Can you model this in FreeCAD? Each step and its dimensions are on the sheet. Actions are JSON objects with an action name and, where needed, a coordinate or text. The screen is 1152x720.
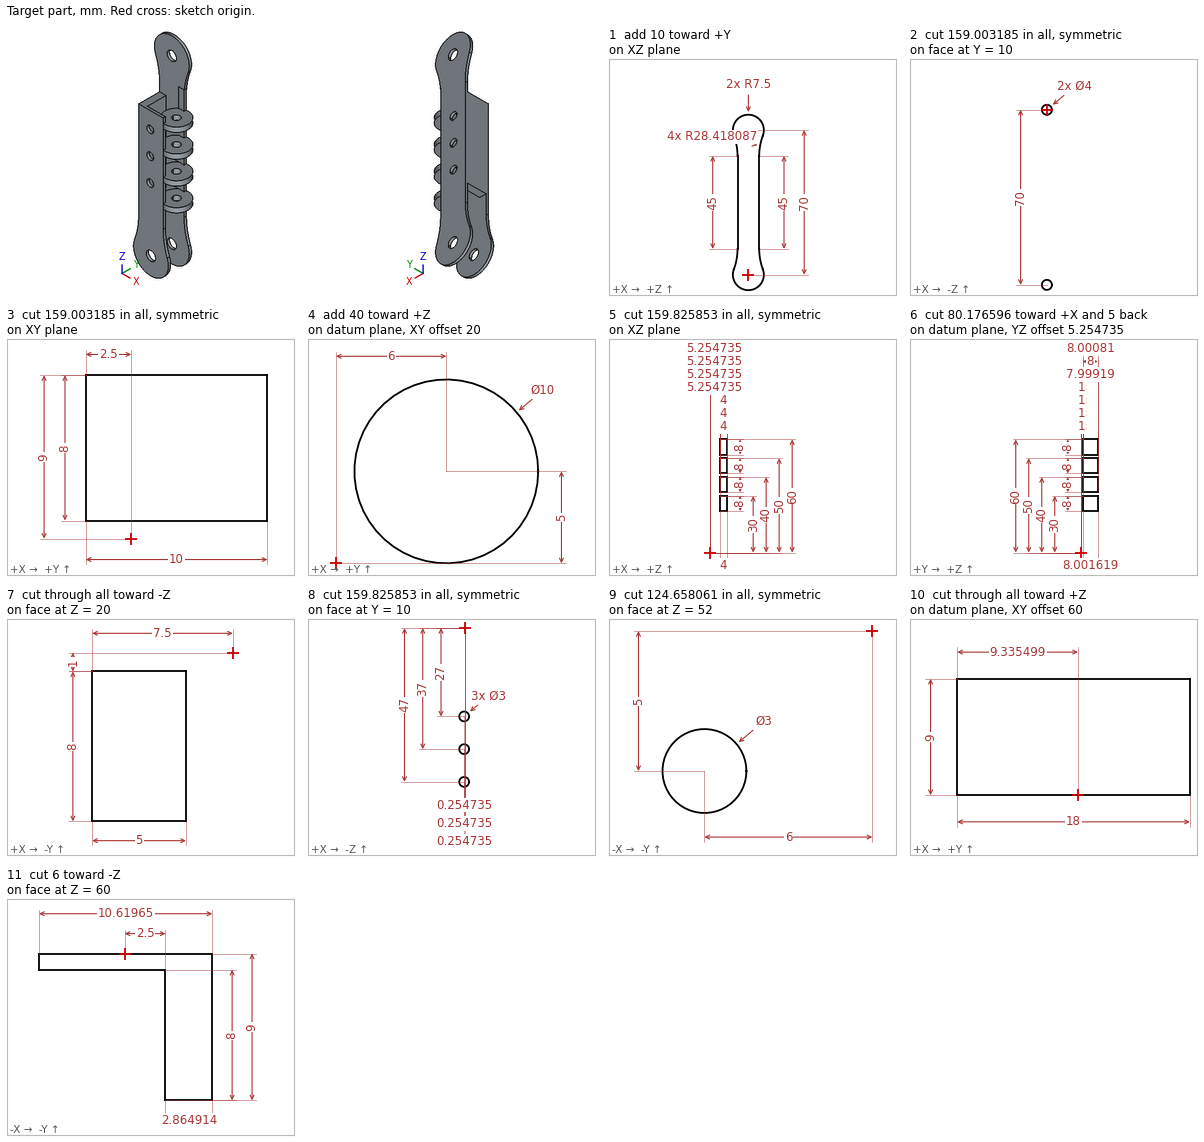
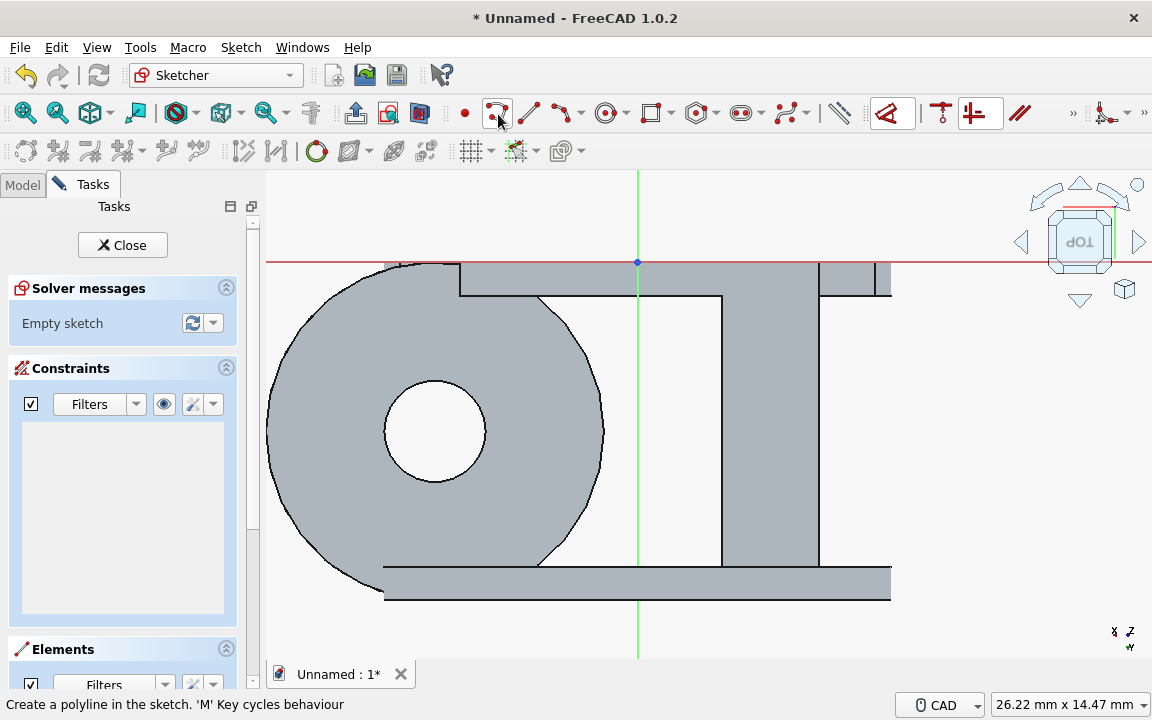
{"action": "left_click", "coordinate": [722, 296]}
{"action": "left_click", "coordinate": [722, 567]}
{"action": "left_click", "coordinate": [819, 567]}
{"action": "left_click", "coordinate": [819, 262]}
{"action": "left_click", "coordinate": [460, 271]}
{"action": "left_click", "coordinate": [460, 296]}
{"action": "left_click", "coordinate": [722, 297]}
{"action": "key", "text": "Escape"}
{"action": "key", "text": "Escape"}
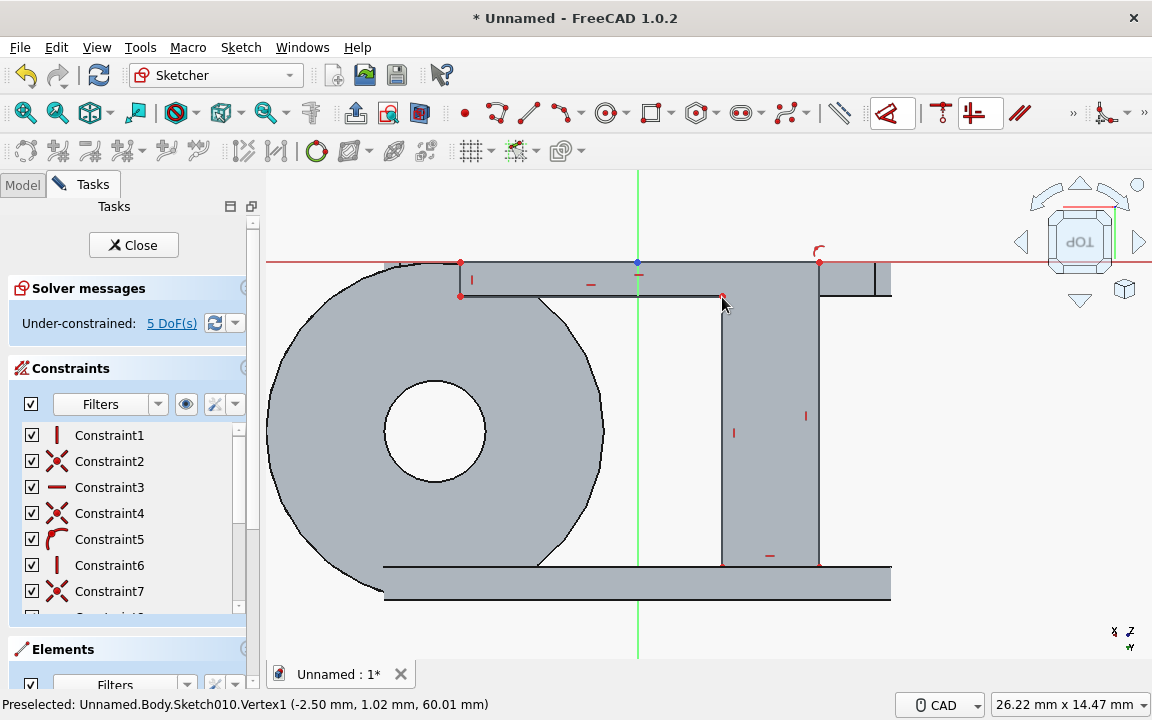
{"action": "left_click", "coordinate": [722, 378]}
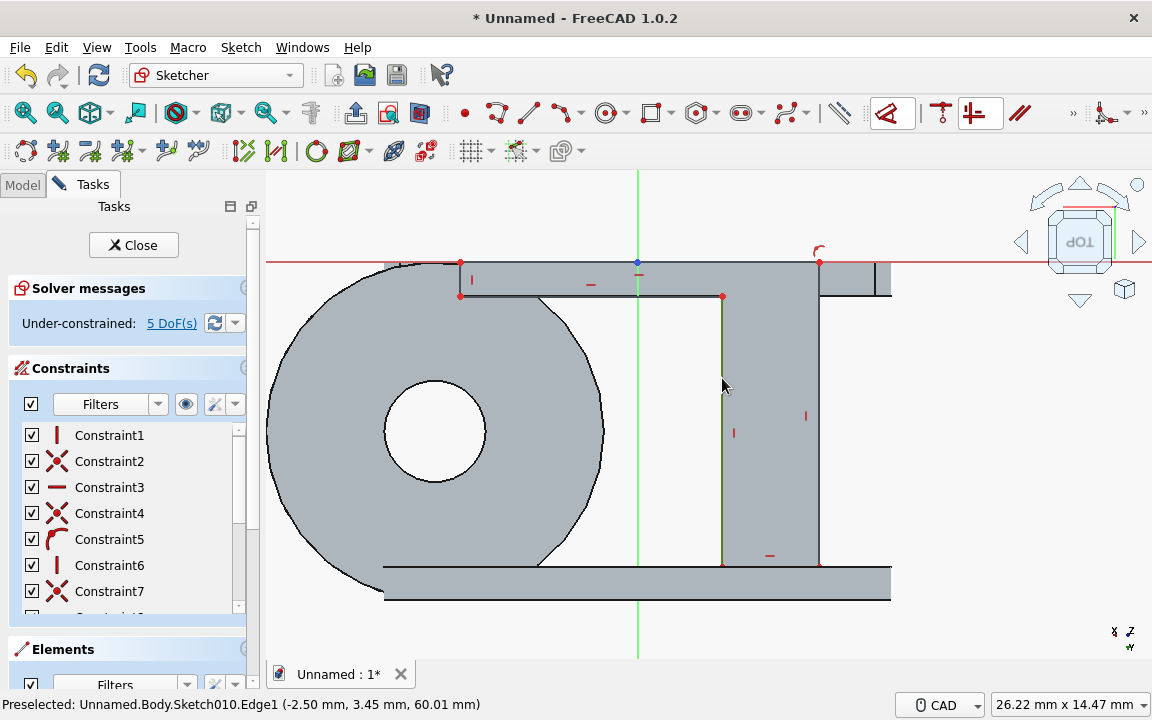
{"action": "left_click", "coordinate": [910, 114]}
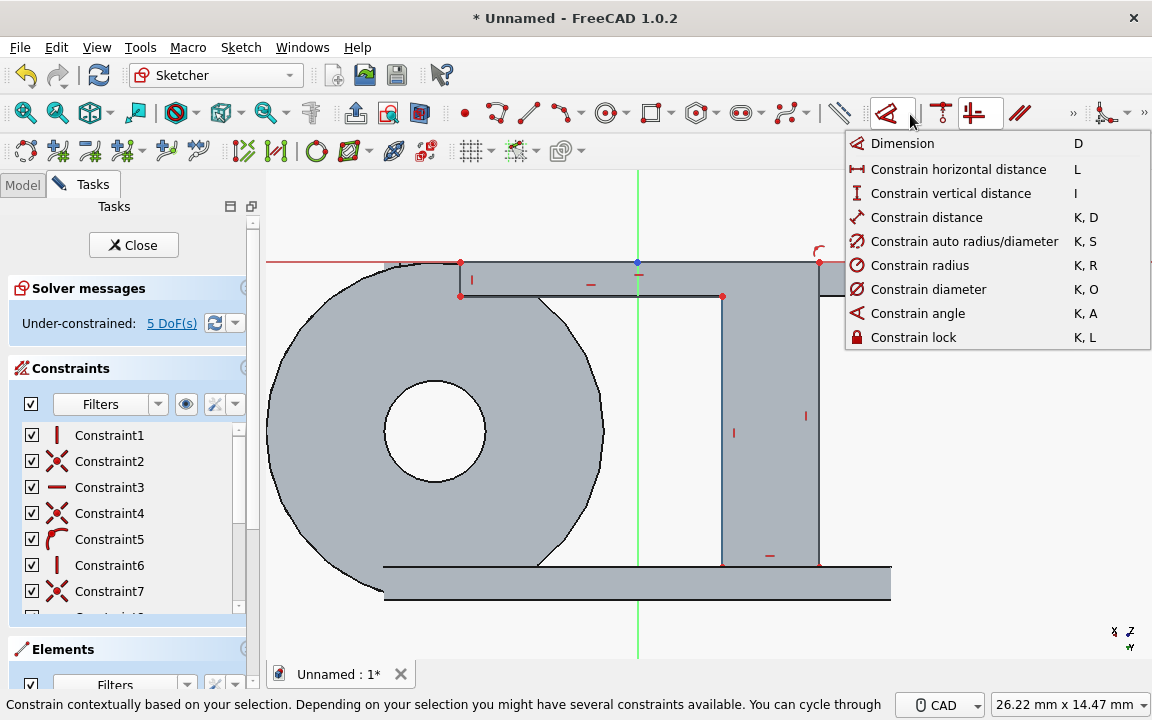
{"action": "left_click", "coordinate": [998, 193]}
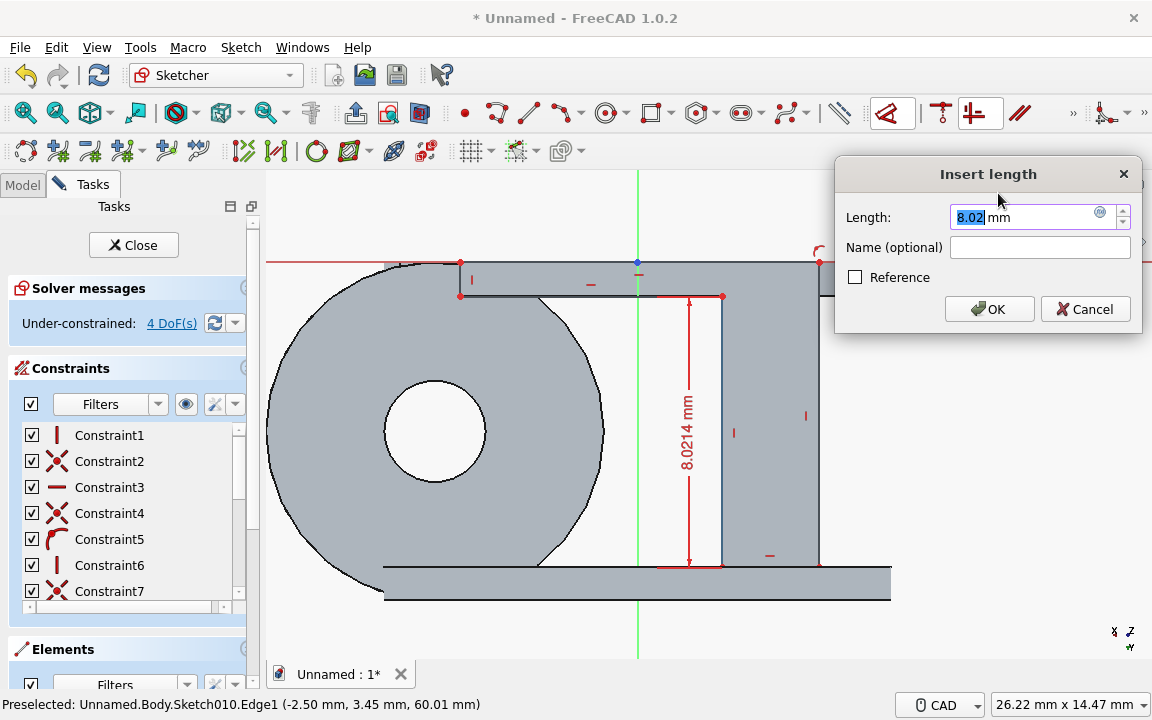
{"action": "type", "text": "8"}
{"action": "key", "text": "Return"}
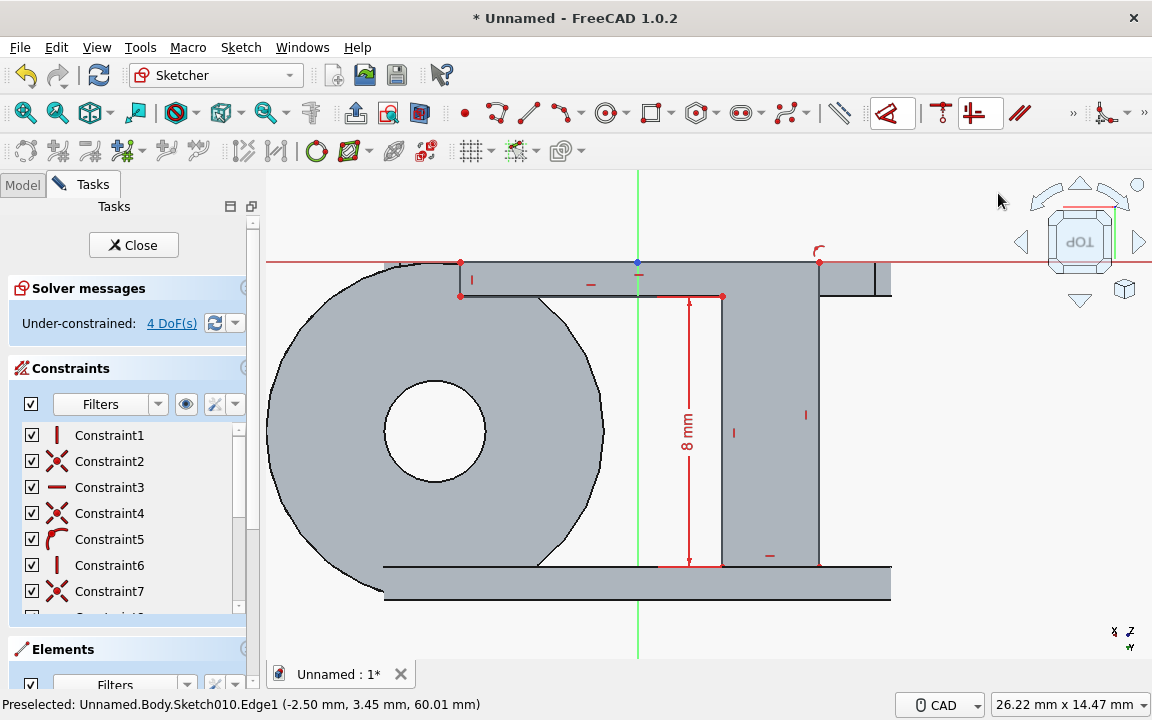
{"action": "left_click", "coordinate": [819, 476]}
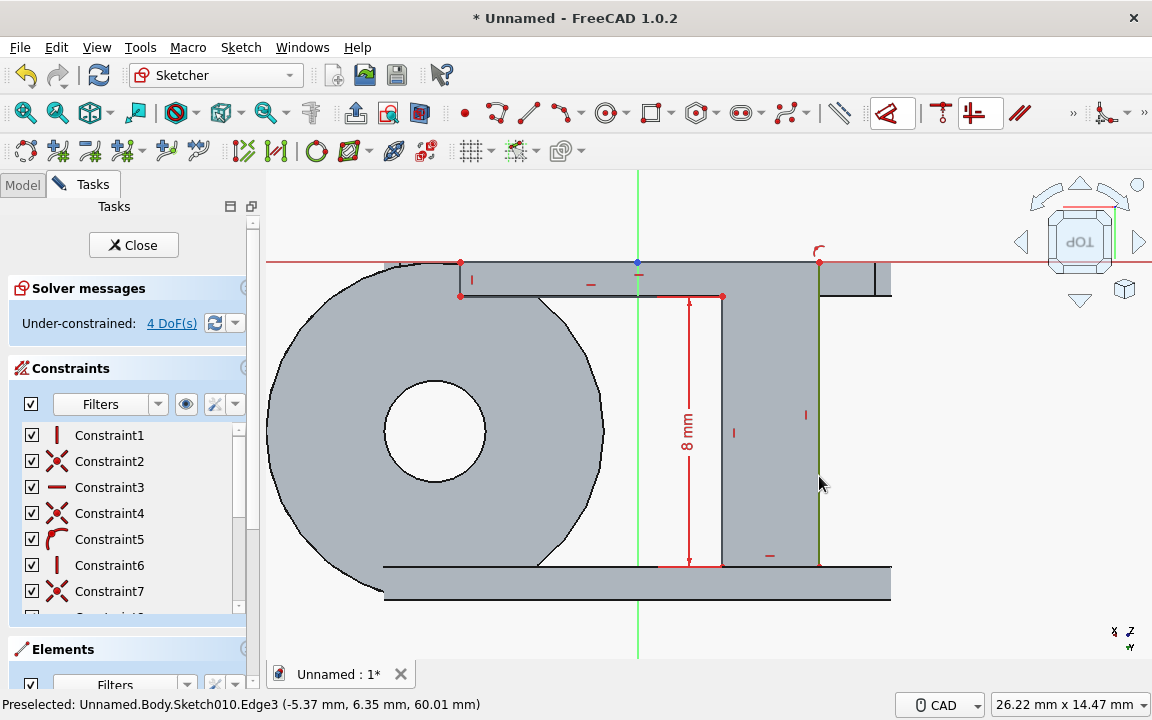
{"action": "left_click", "coordinate": [910, 114]}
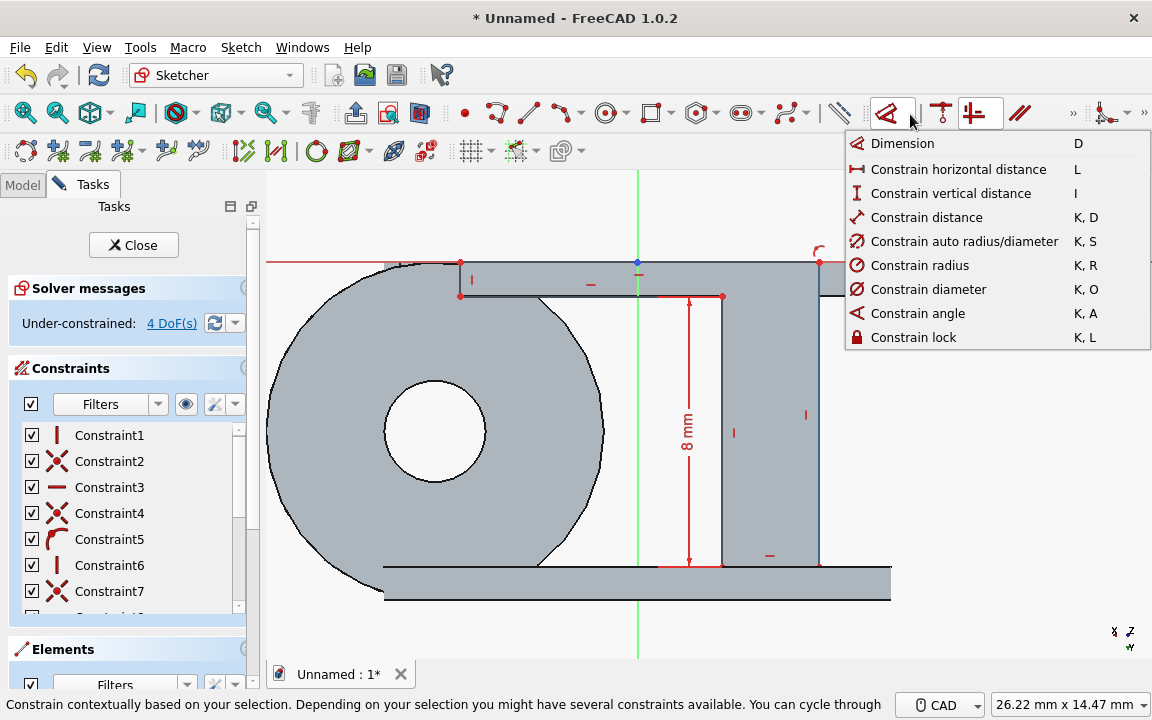
{"action": "left_click", "coordinate": [998, 193]}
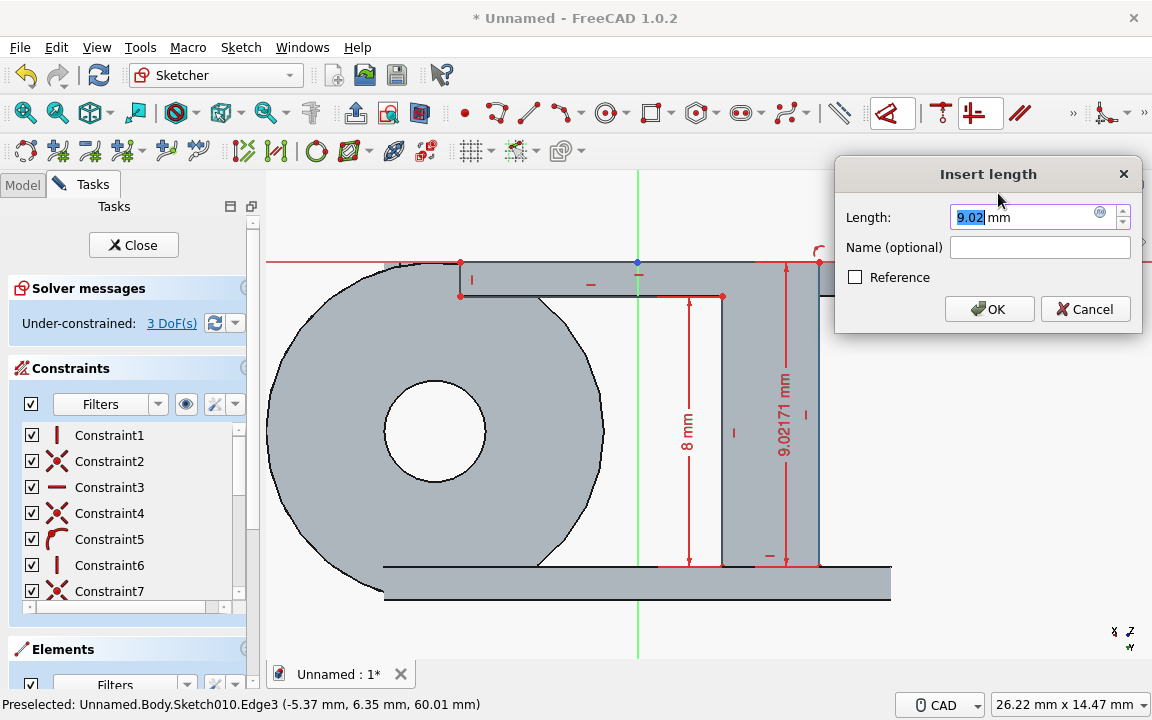
{"action": "type", "text": "9"}
{"action": "key", "text": "Return"}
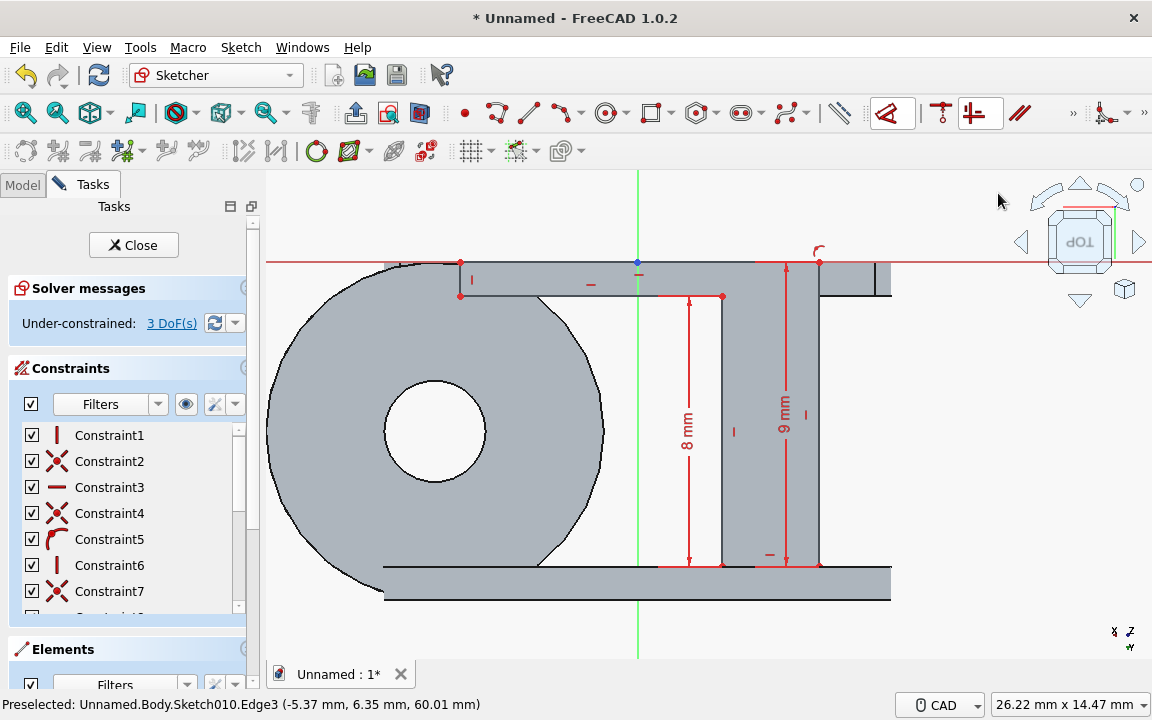
{"action": "left_click", "coordinate": [722, 296]}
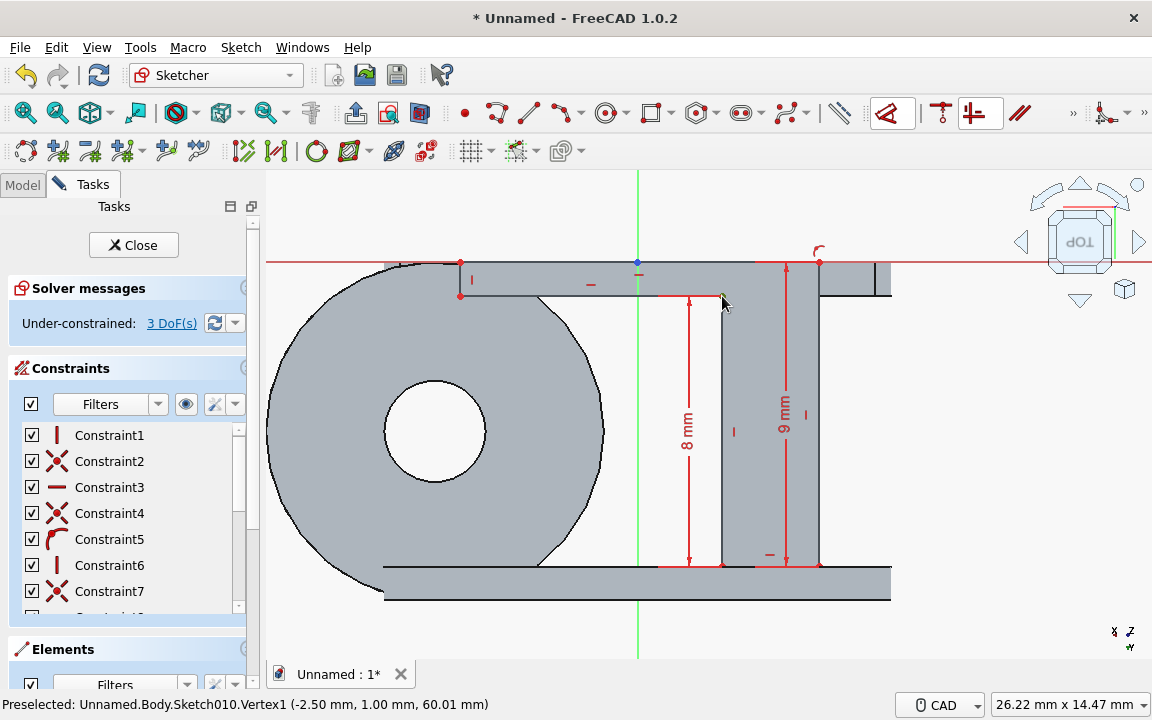
{"action": "key", "text": "l"}